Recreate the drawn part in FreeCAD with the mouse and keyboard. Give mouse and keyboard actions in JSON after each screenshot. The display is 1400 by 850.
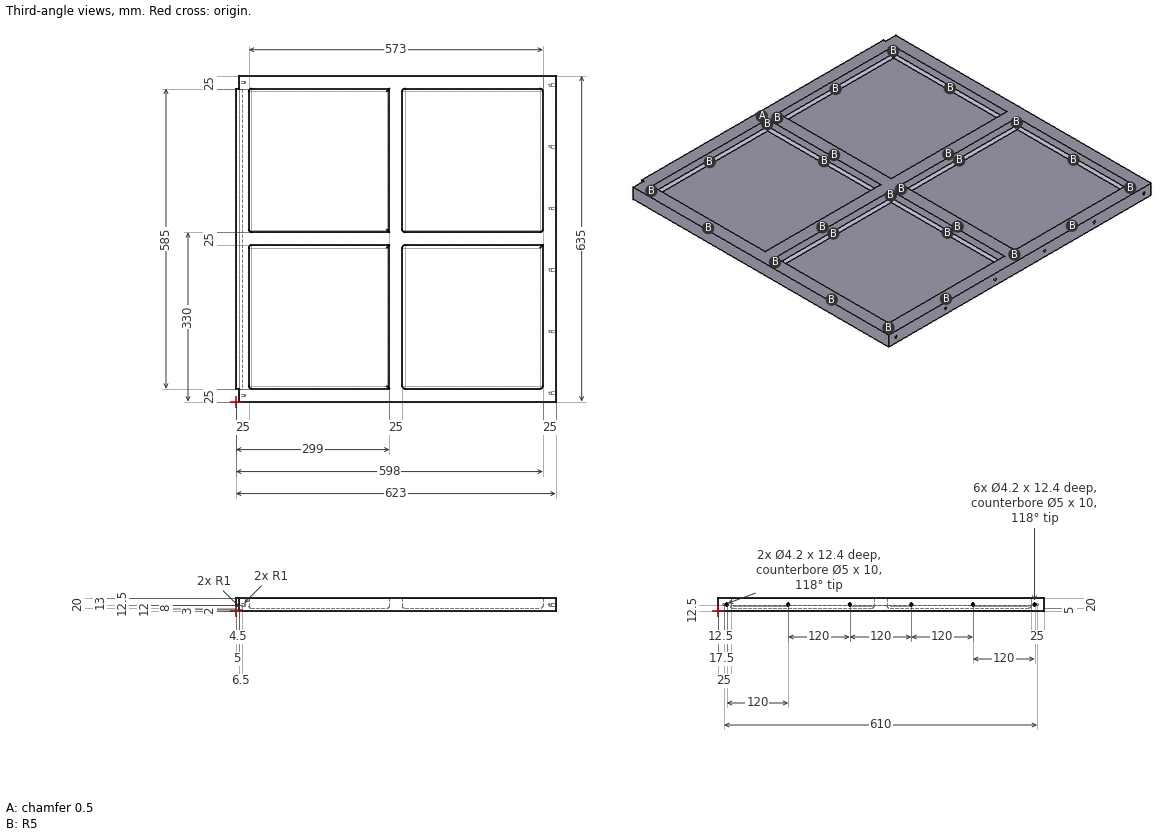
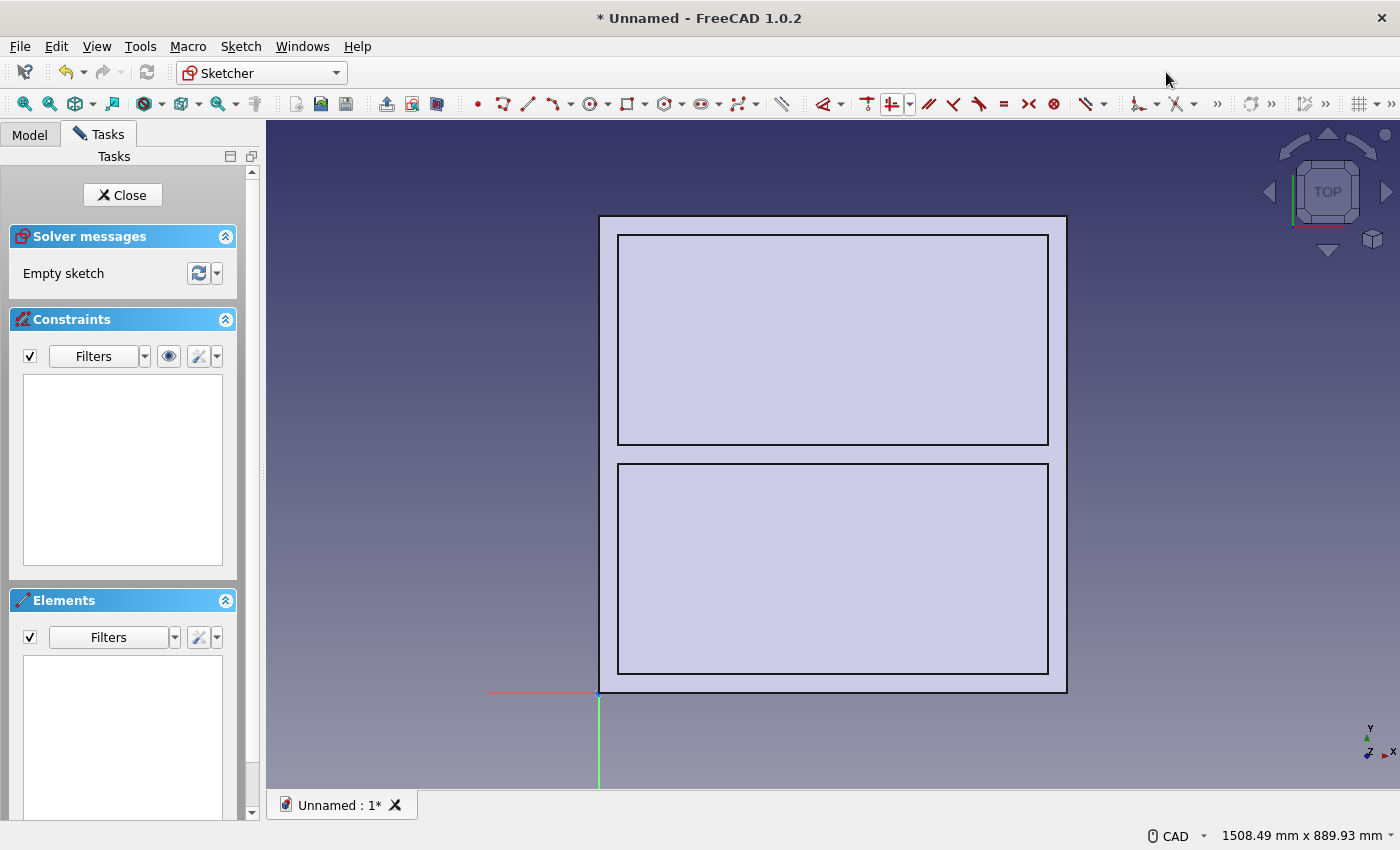
{"action": "left_click", "coordinate": [437, 104]}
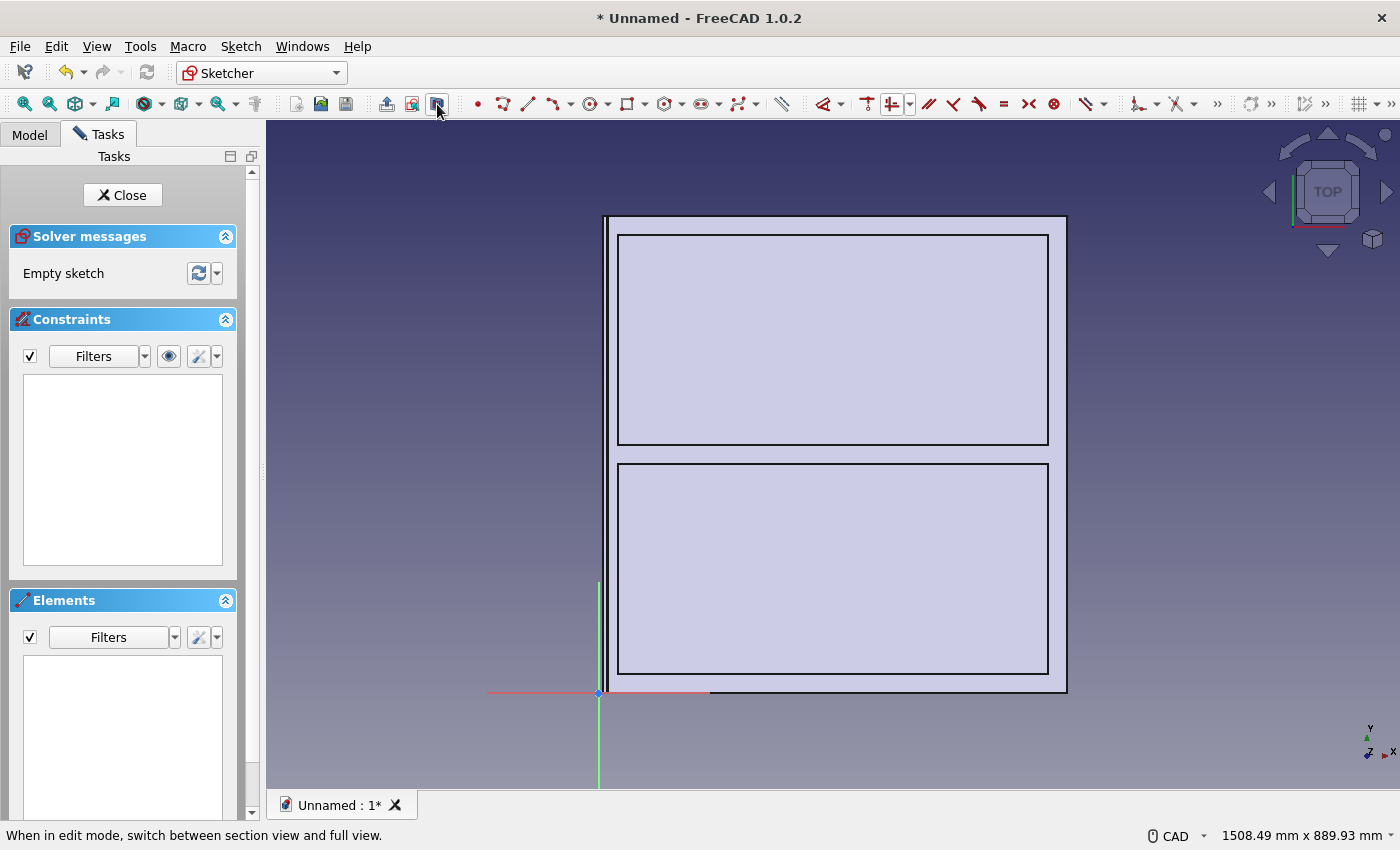
{"action": "key", "text": "g r"}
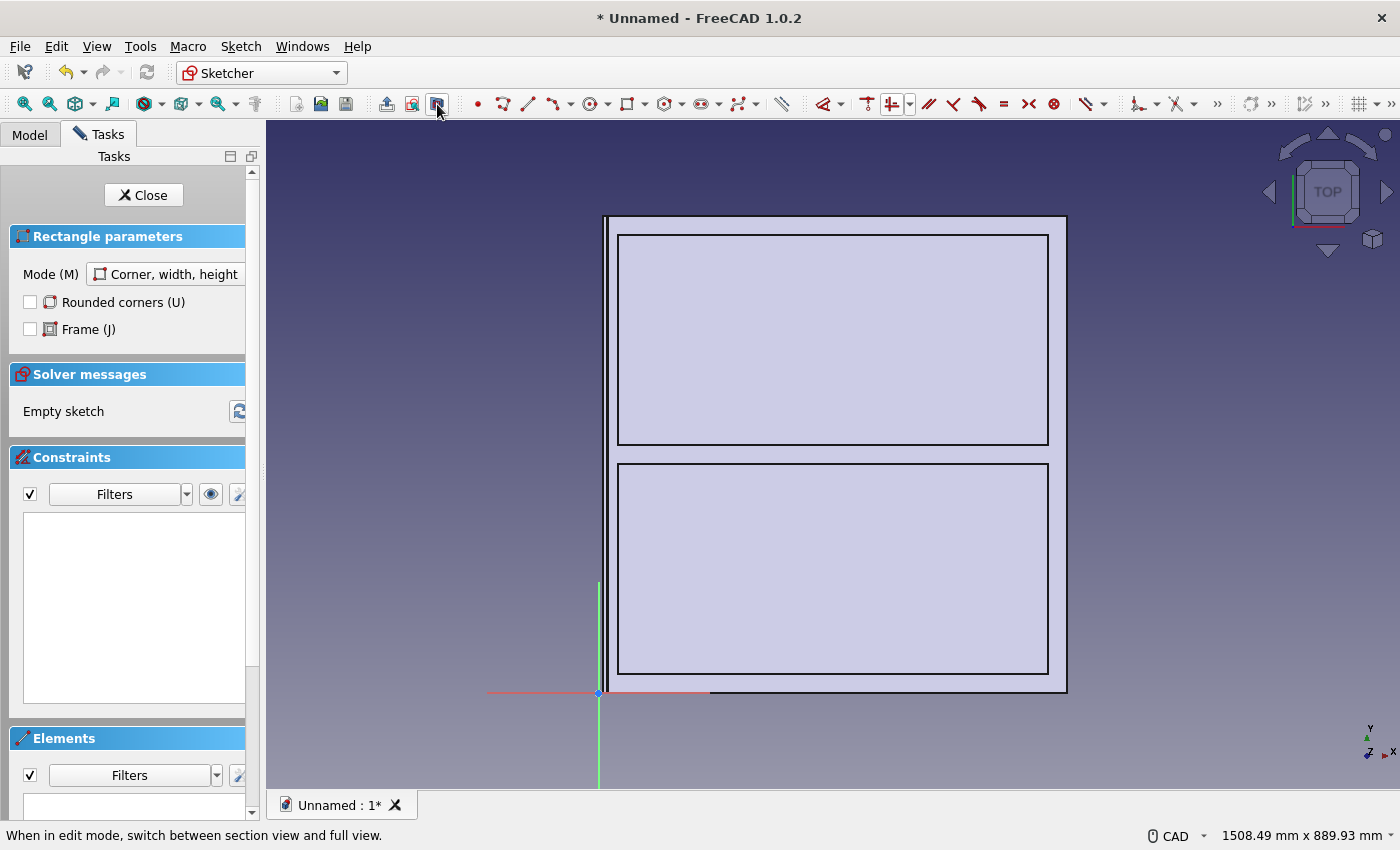
{"action": "left_click", "coordinate": [824, 235]}
{"action": "left_click", "coordinate": [842, 674]}
{"action": "key", "text": "Escape"}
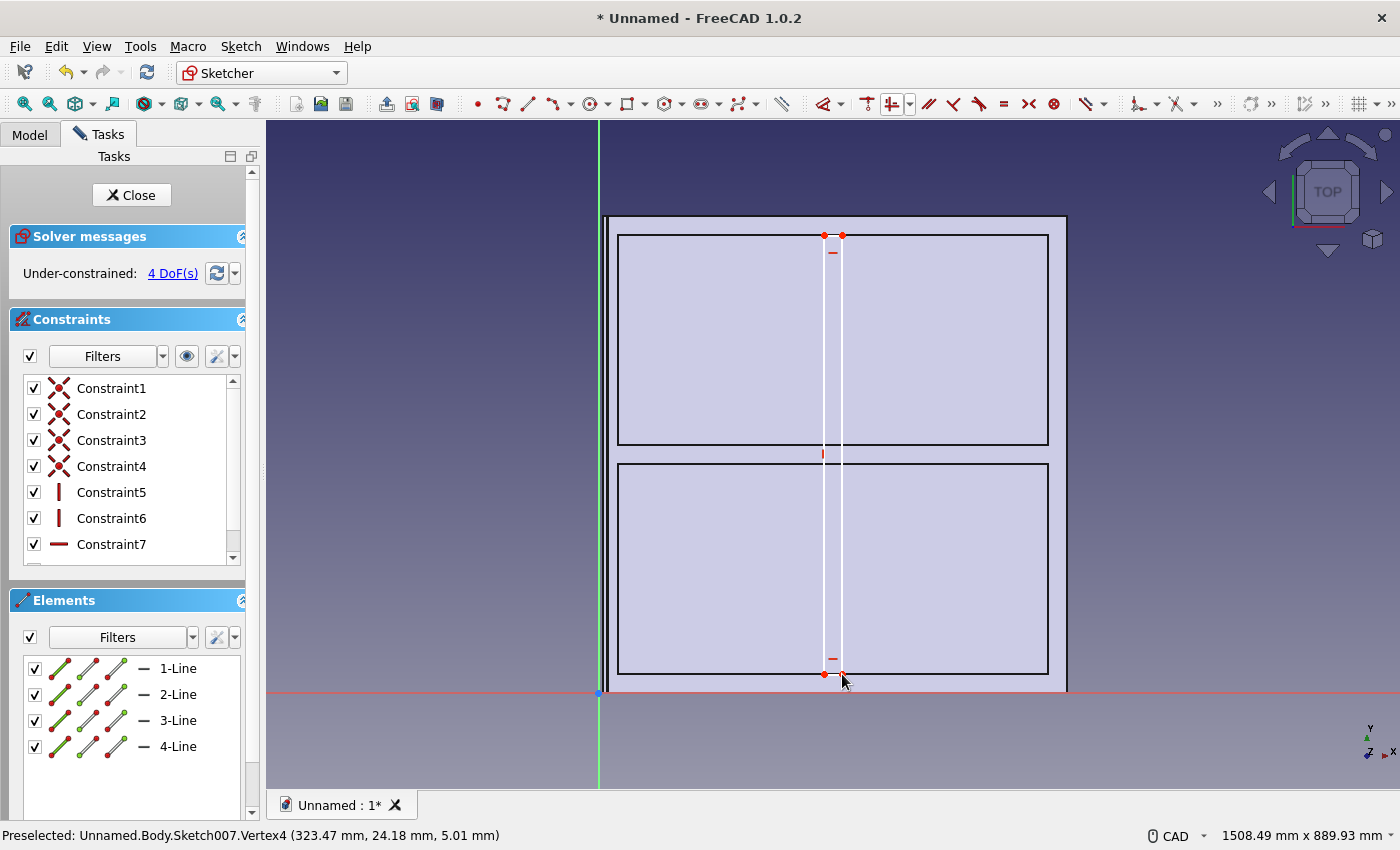
{"action": "left_click", "coordinate": [822, 104]}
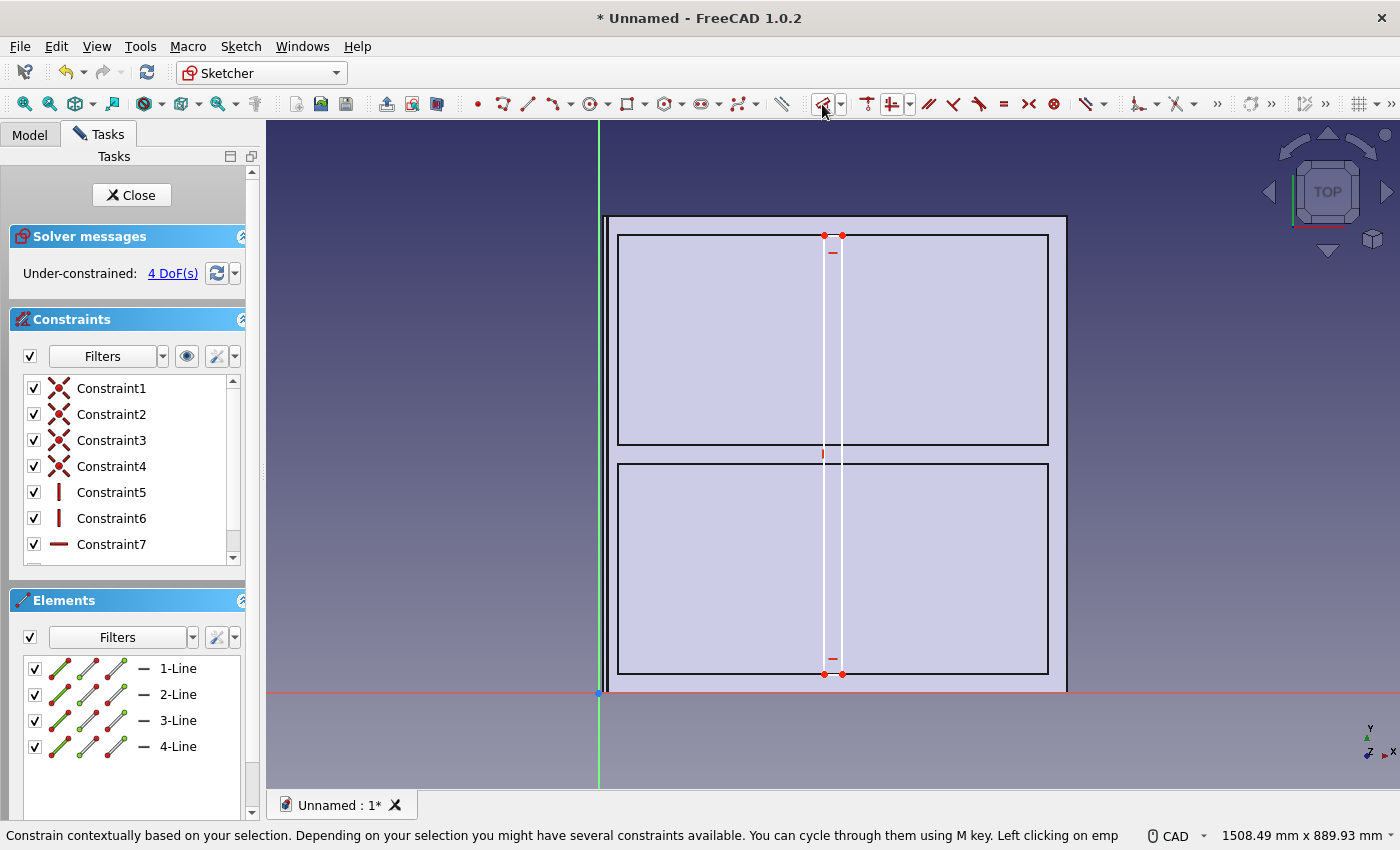
{"action": "scroll", "coordinate": [833, 675], "scroll_direction": "up", "scroll_amount": 4}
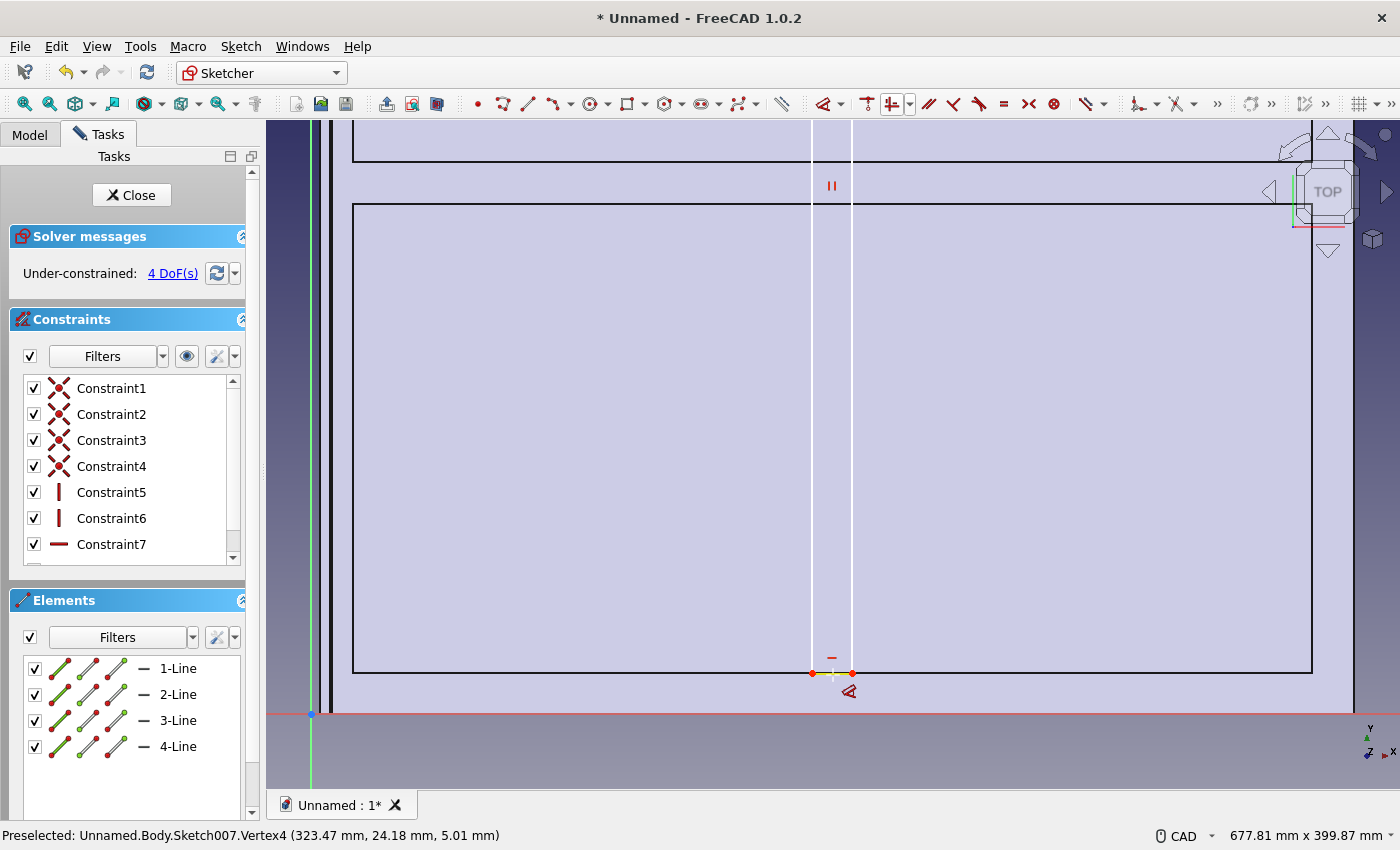
{"action": "left_click", "coordinate": [832, 674]}
{"action": "left_click", "coordinate": [832, 640]}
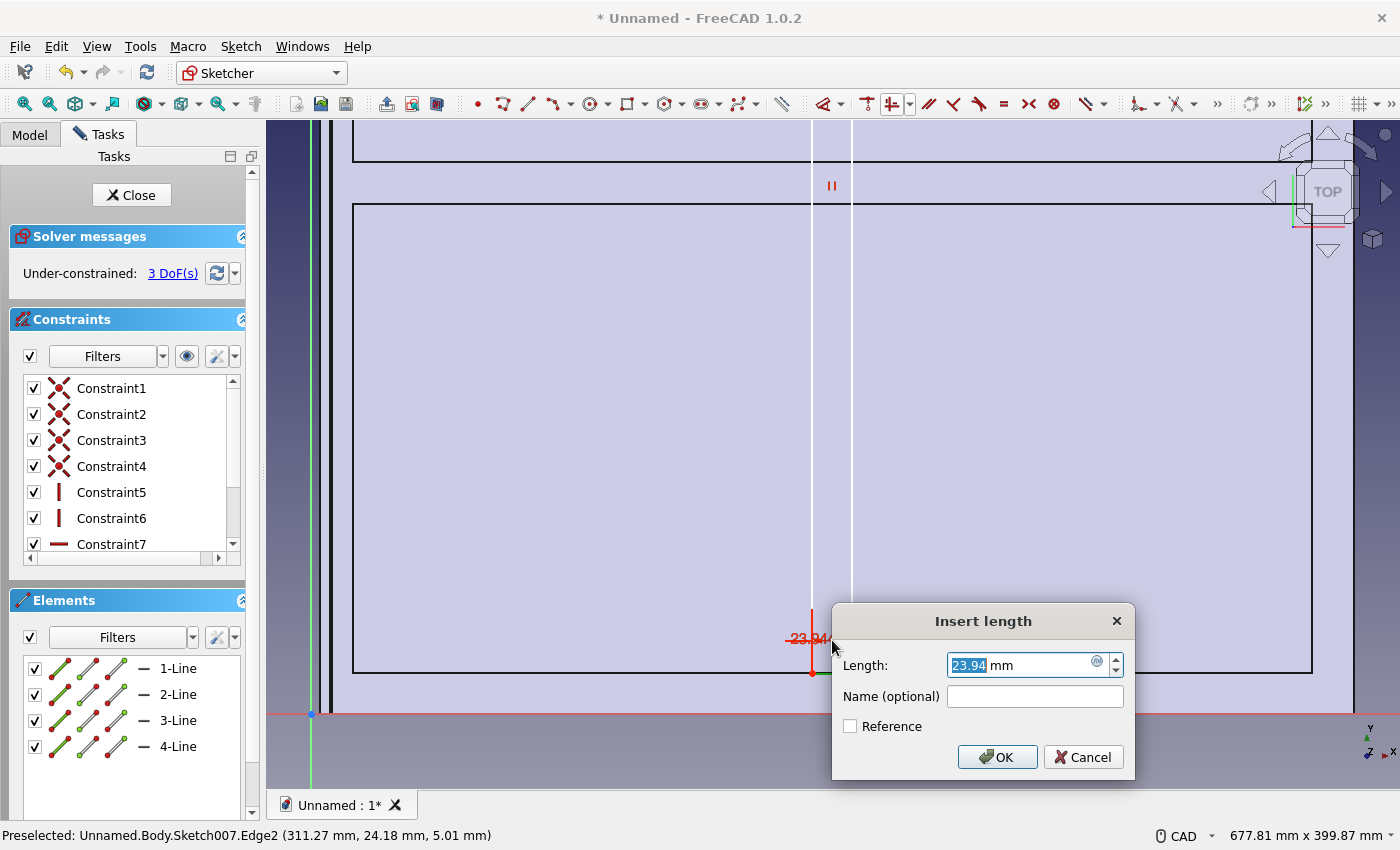
{"action": "type", "text": "25"}
{"action": "key", "text": "Return"}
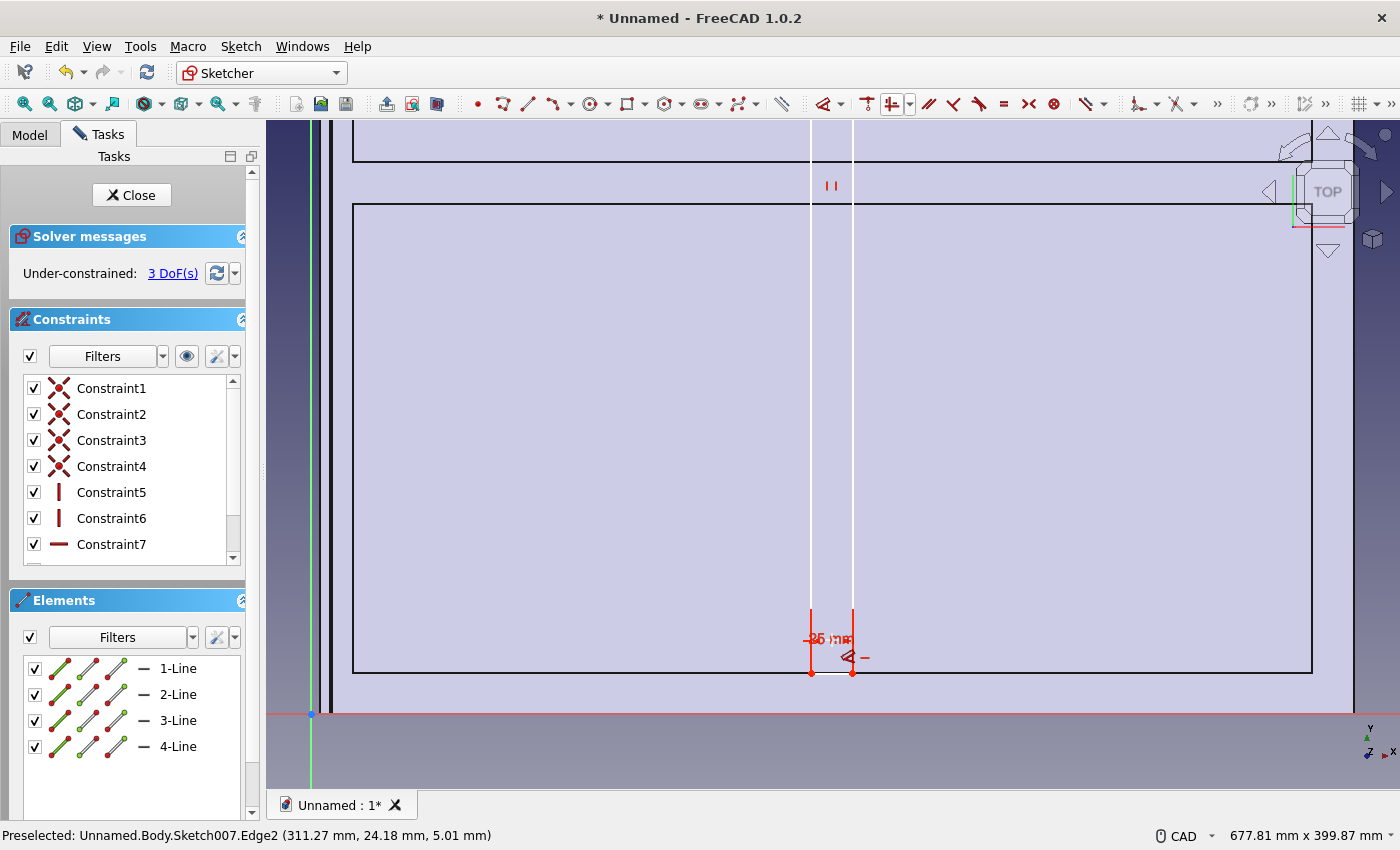
{"action": "left_click", "coordinate": [811, 381]}
{"action": "left_click", "coordinate": [777, 411]}